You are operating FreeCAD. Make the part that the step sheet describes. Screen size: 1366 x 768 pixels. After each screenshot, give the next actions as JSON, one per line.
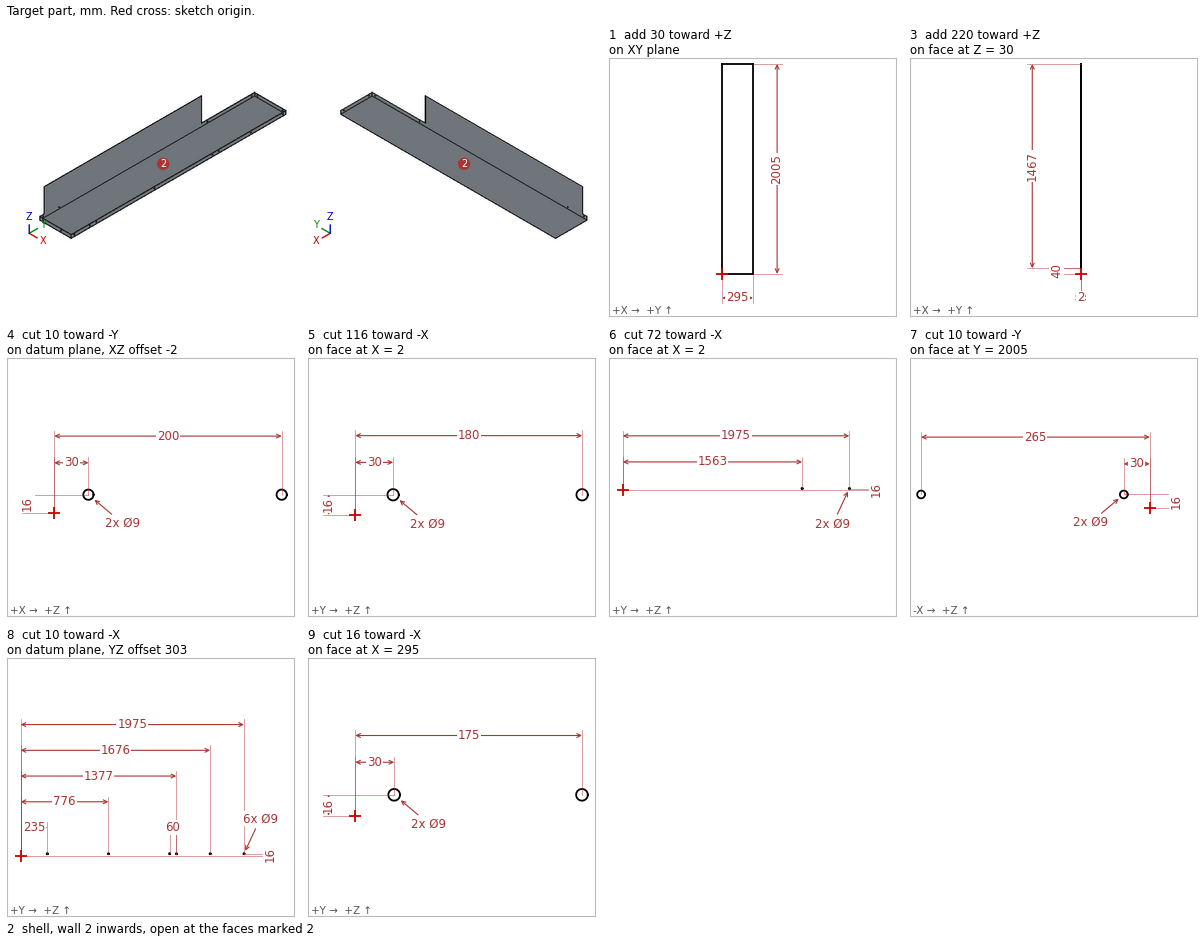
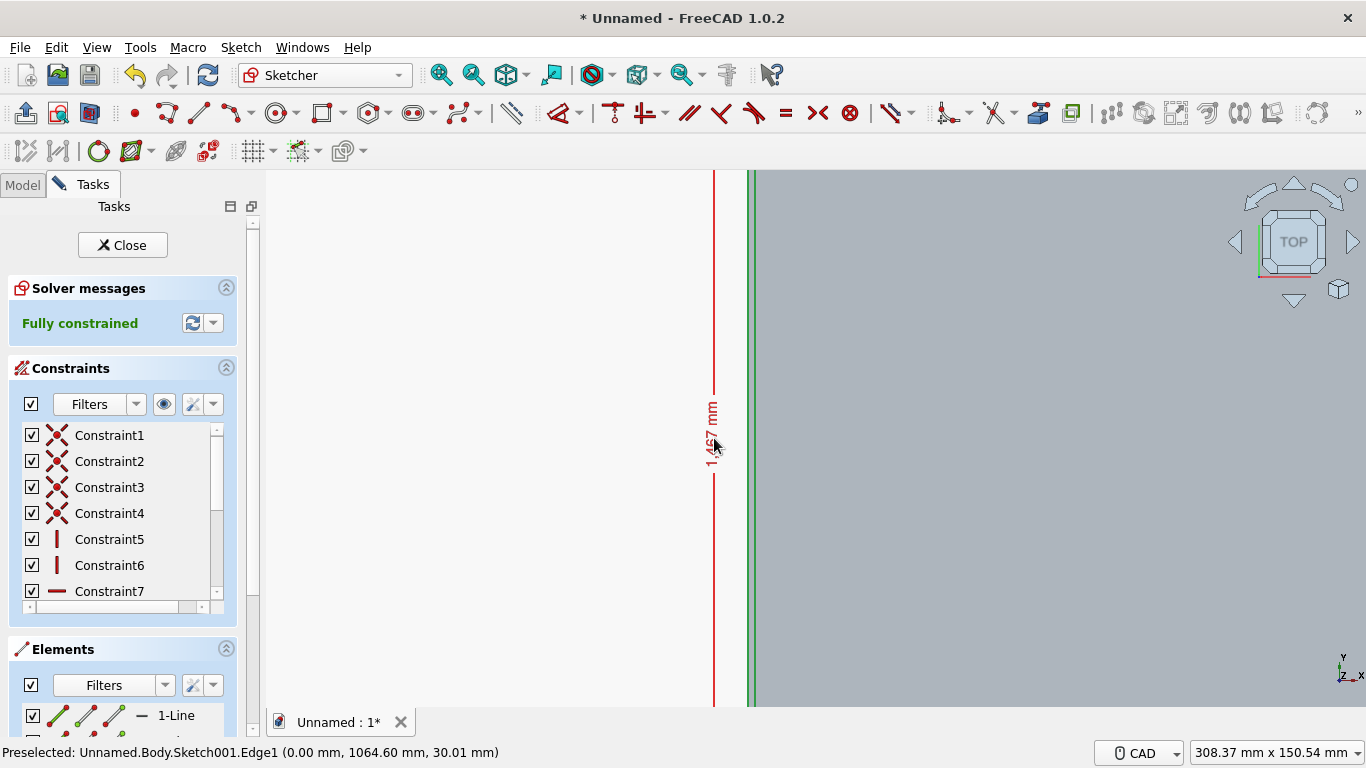
{"action": "left_click", "coordinate": [123, 245]}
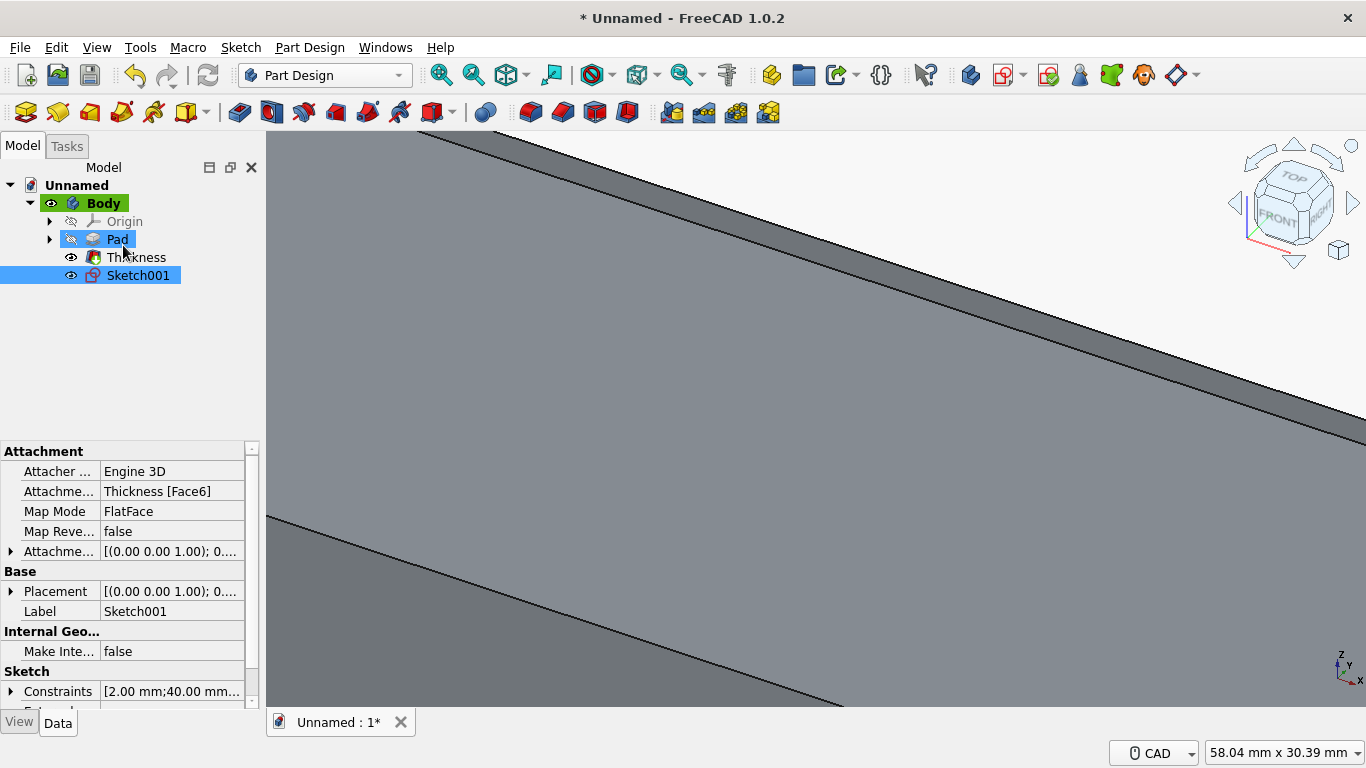
{"action": "left_click", "coordinate": [26, 112]}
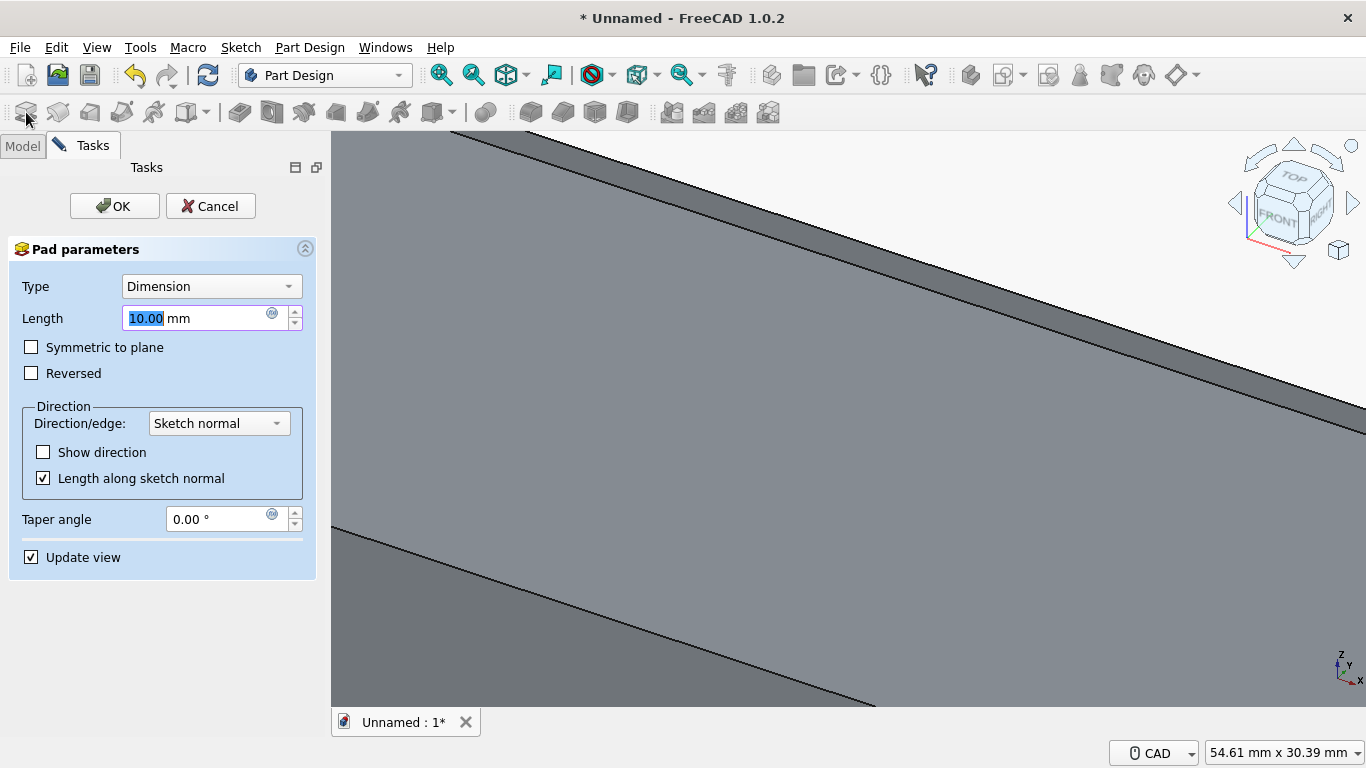
{"action": "type", "text": "220"}
{"action": "key", "text": "Tab"}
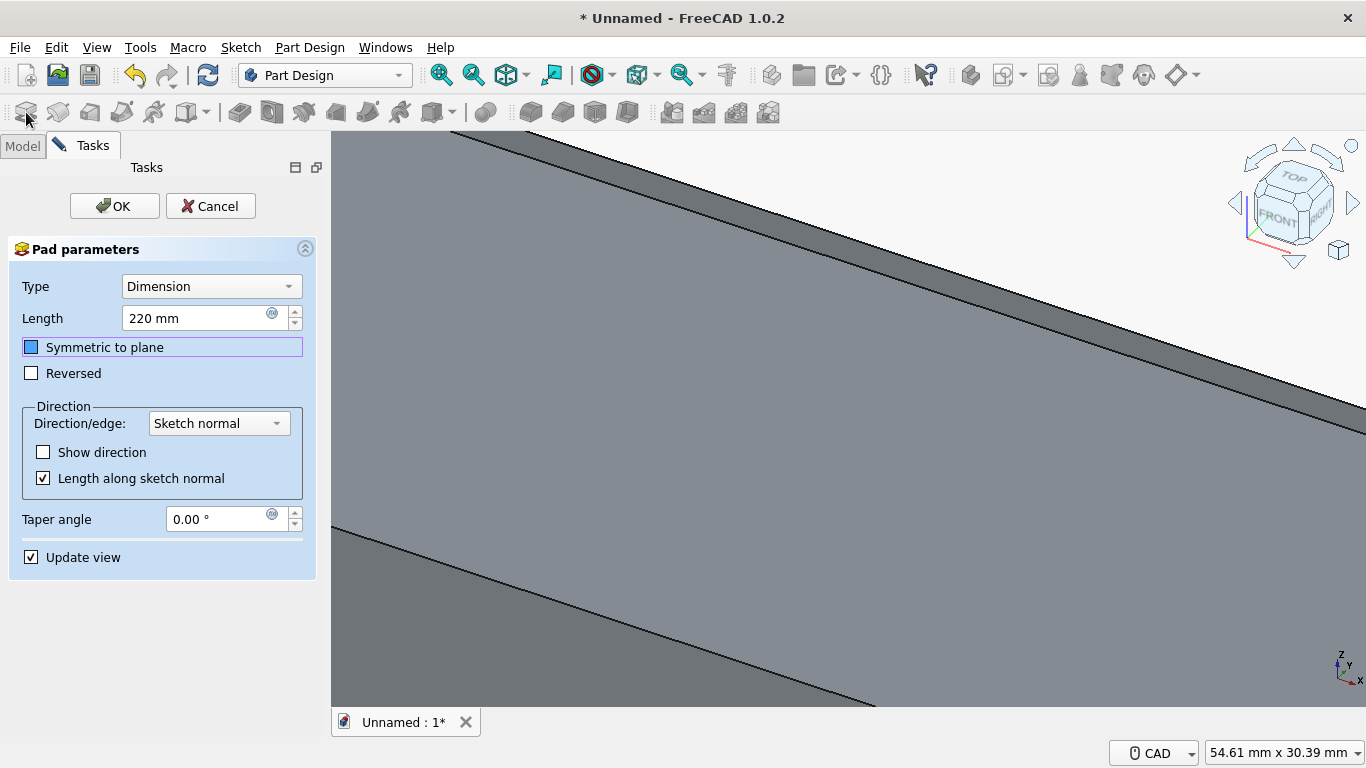
{"action": "left_click", "coordinate": [115, 206]}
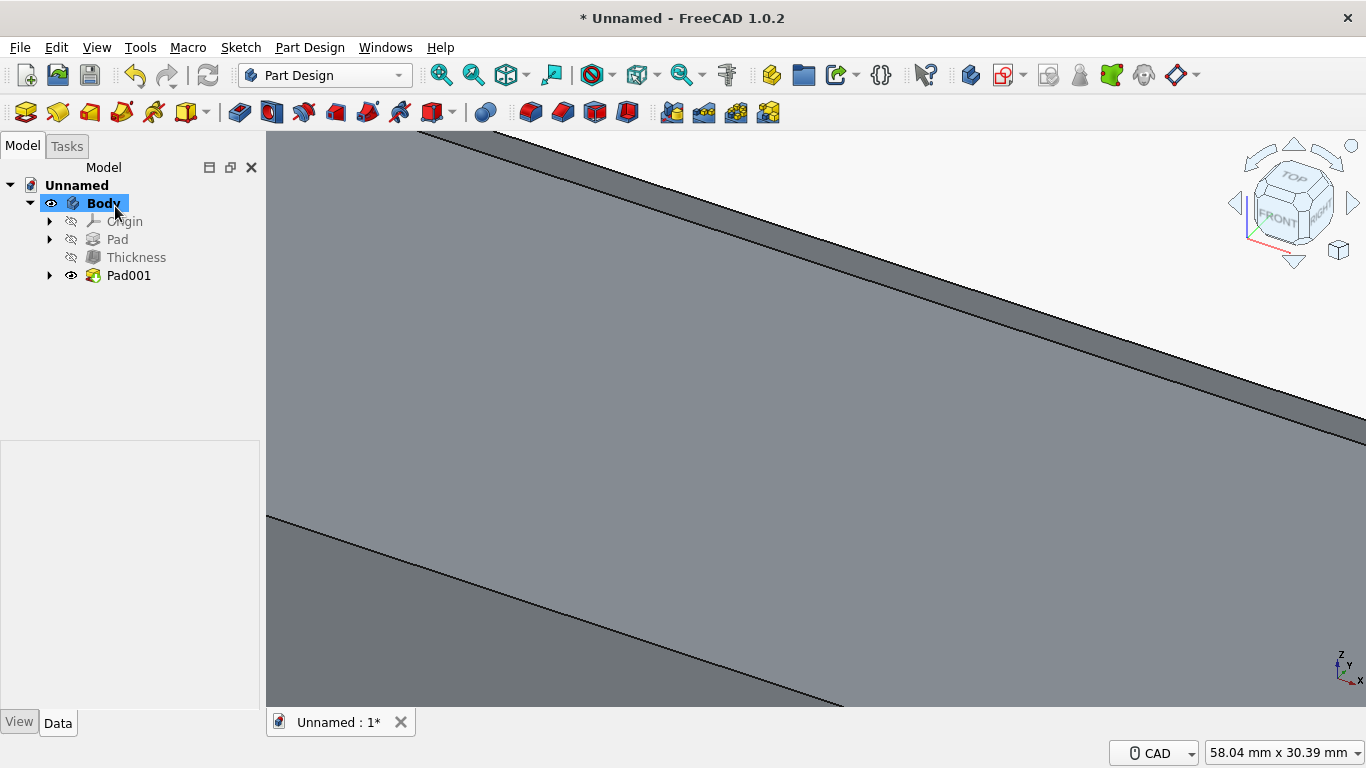
{"action": "key", "text": "v f"}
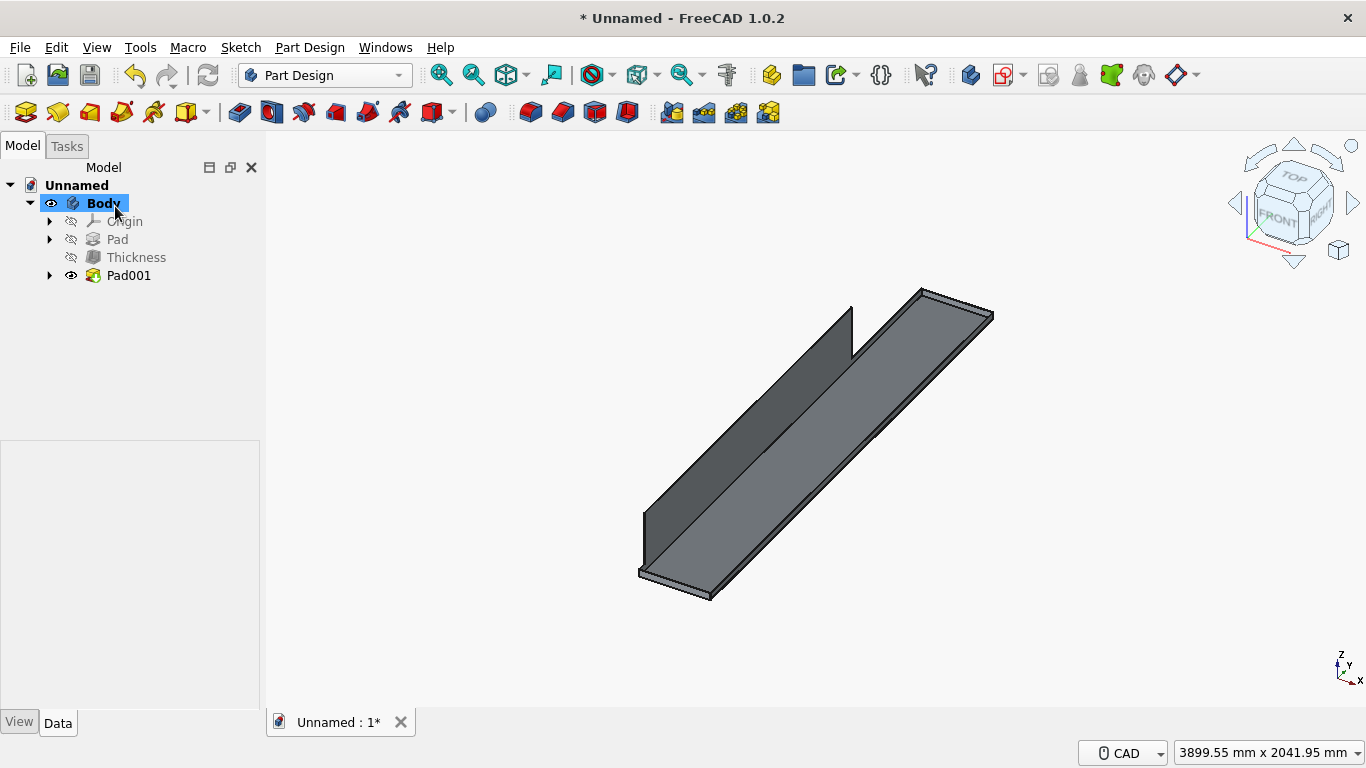
{"action": "left_click", "coordinate": [50, 221]}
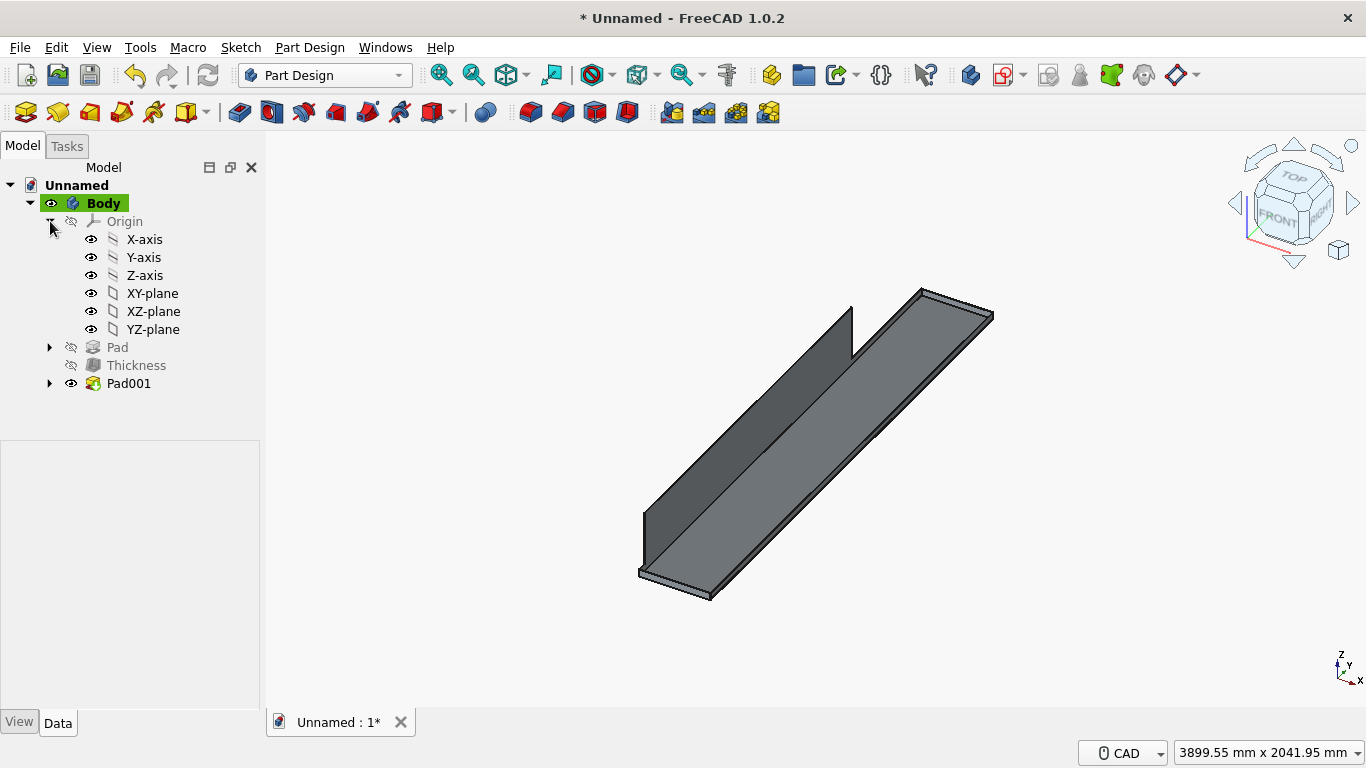
{"action": "left_click", "coordinate": [136, 311]}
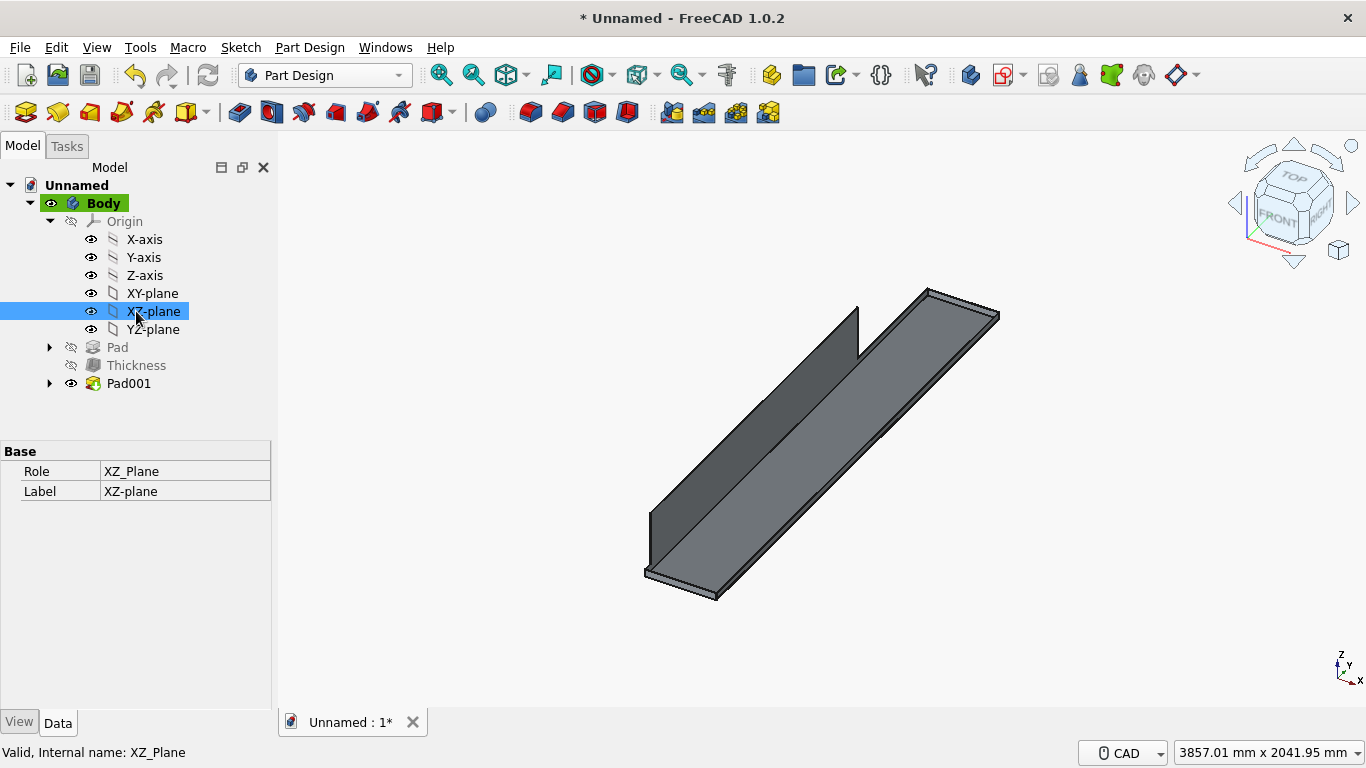
{"action": "left_click", "coordinate": [1176, 76]}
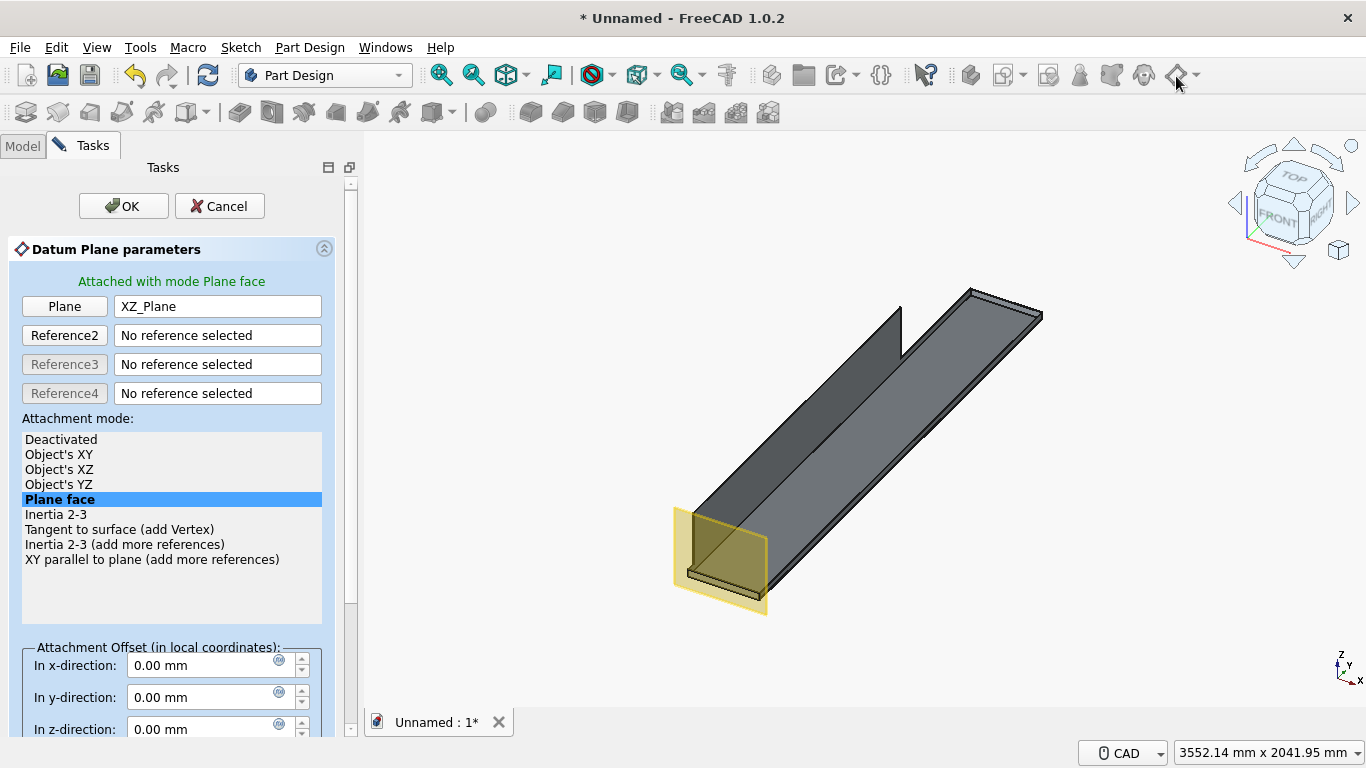
{"action": "scroll", "coordinate": [351, 456], "scroll_direction": "down", "scroll_amount": 2}